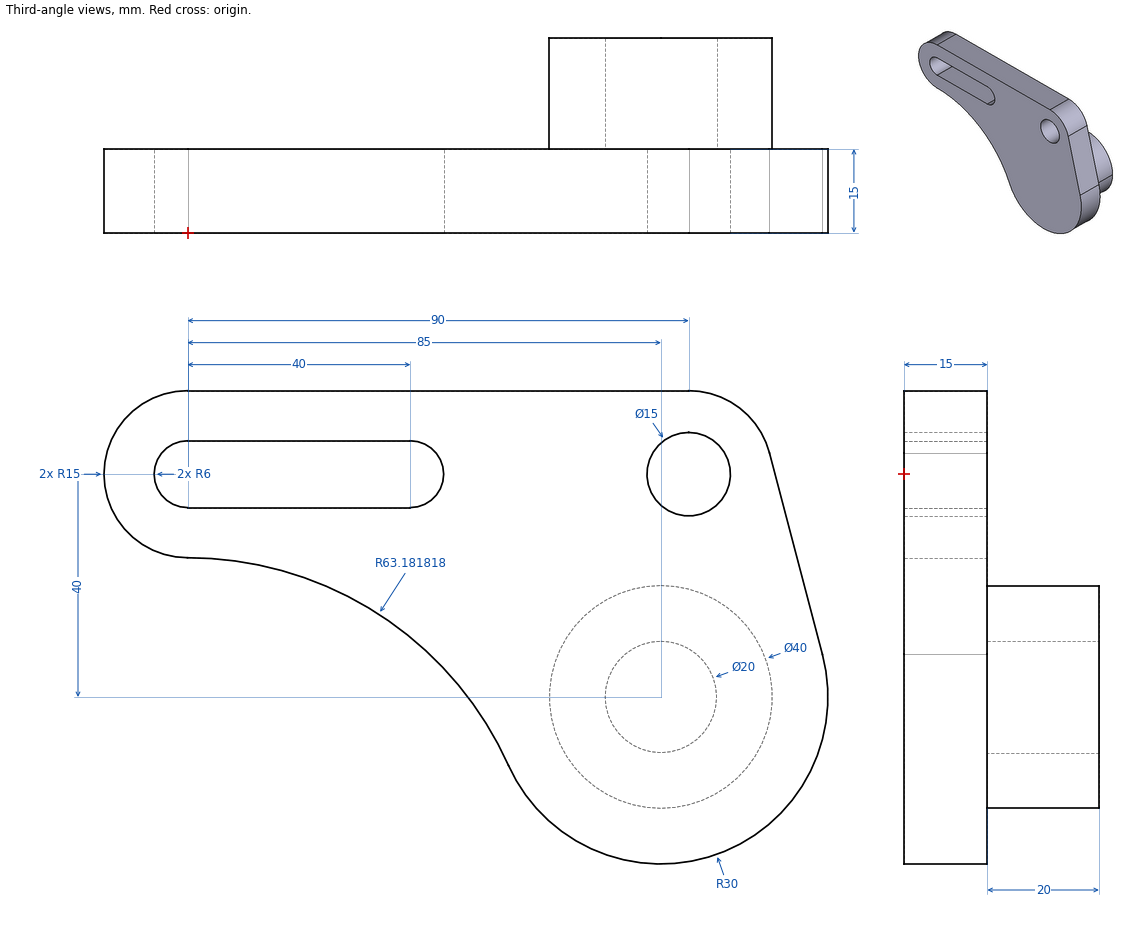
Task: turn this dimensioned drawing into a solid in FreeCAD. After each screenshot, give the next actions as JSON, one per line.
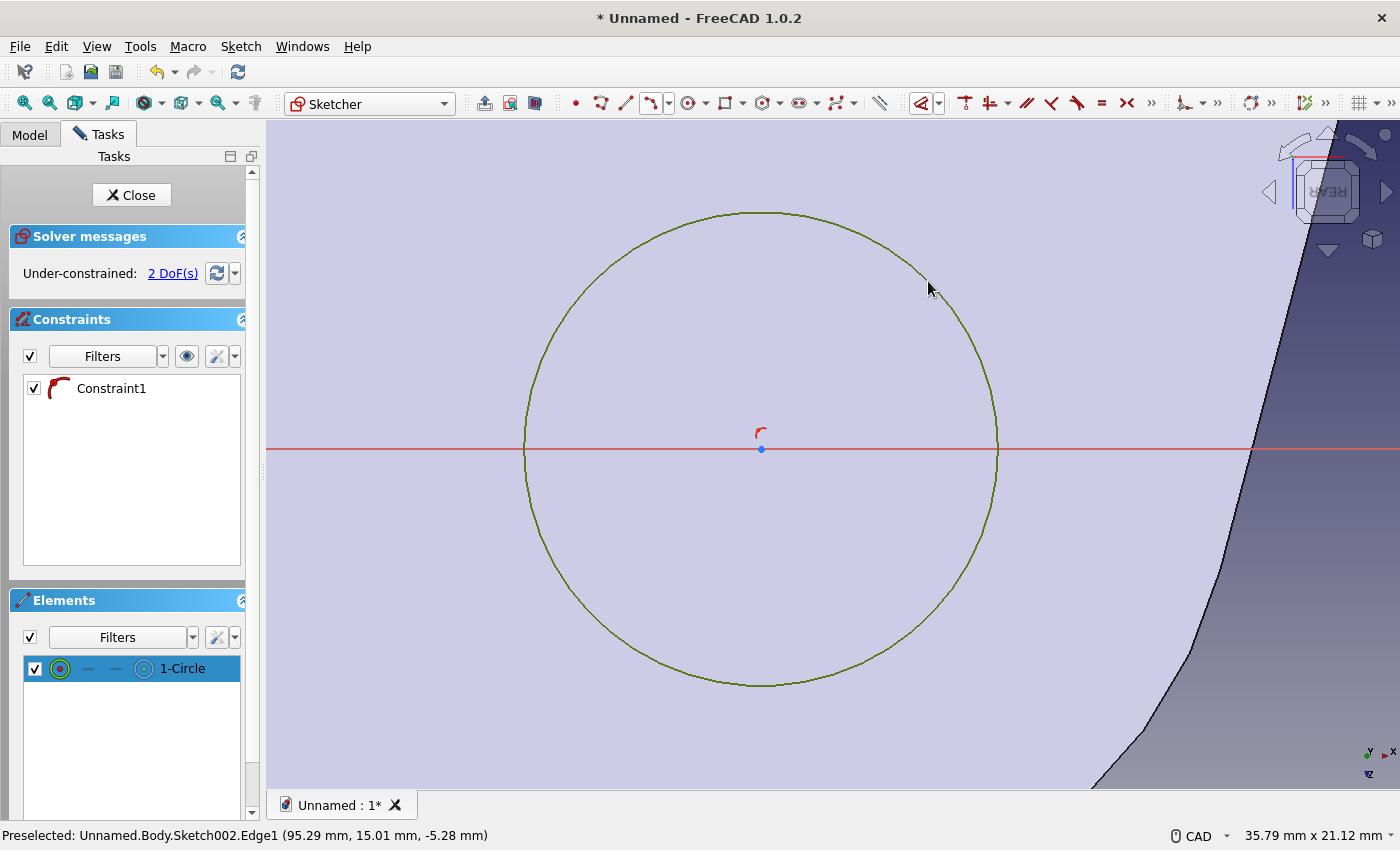
{"action": "left_click", "coordinate": [938, 104]}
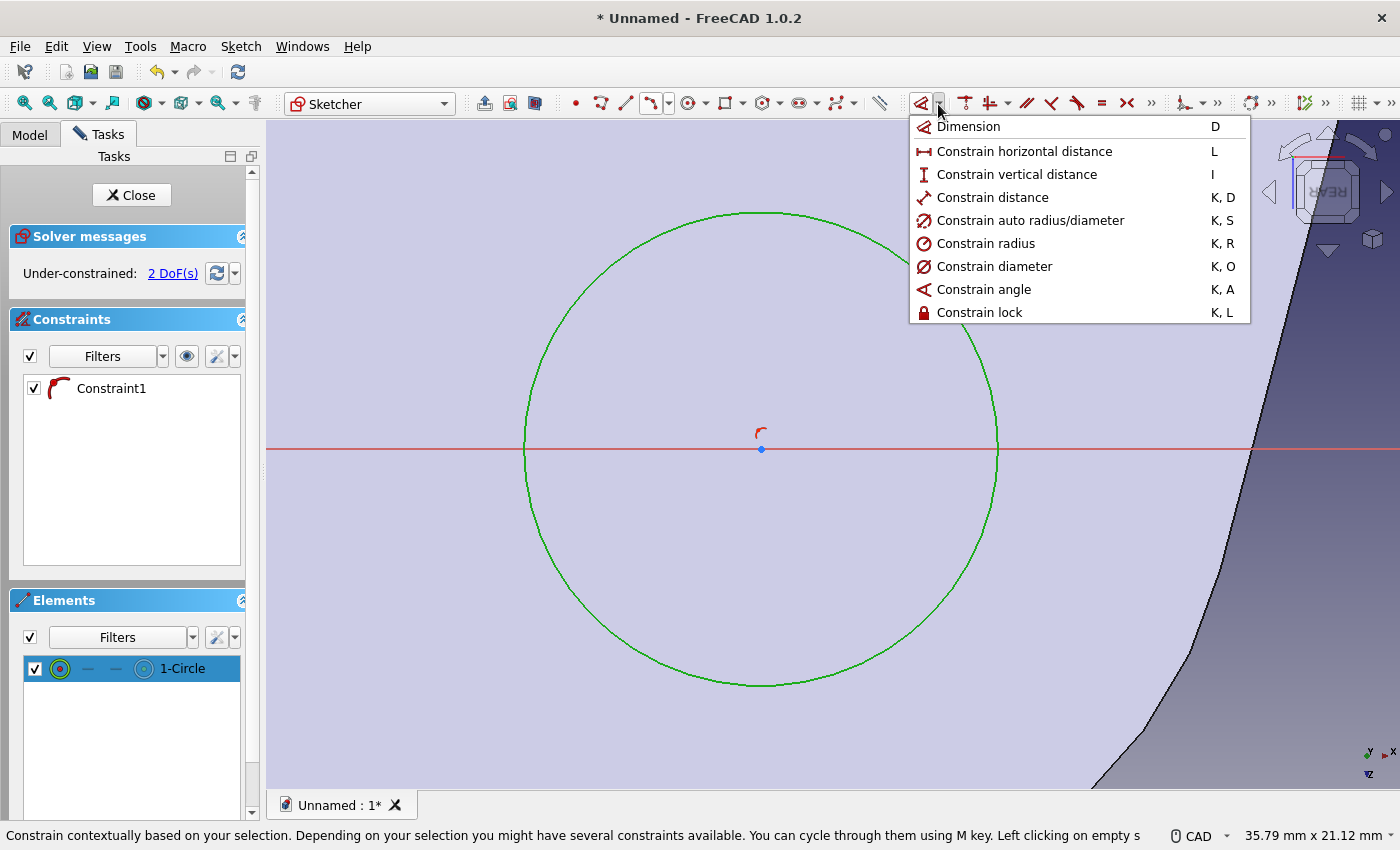
{"action": "left_click", "coordinate": [1080, 266]}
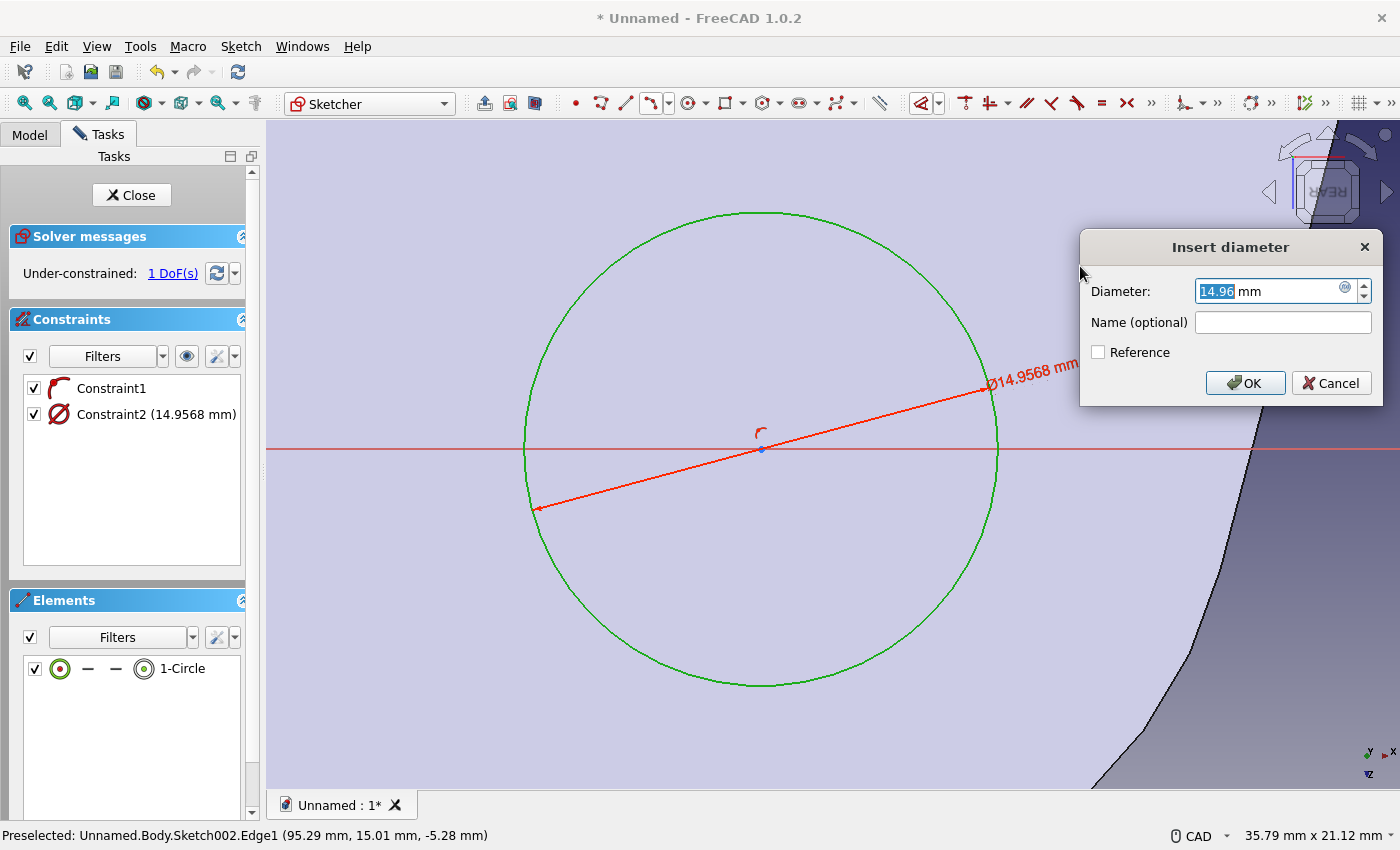
{"action": "type", "text": "15"}
{"action": "key", "text": "Return"}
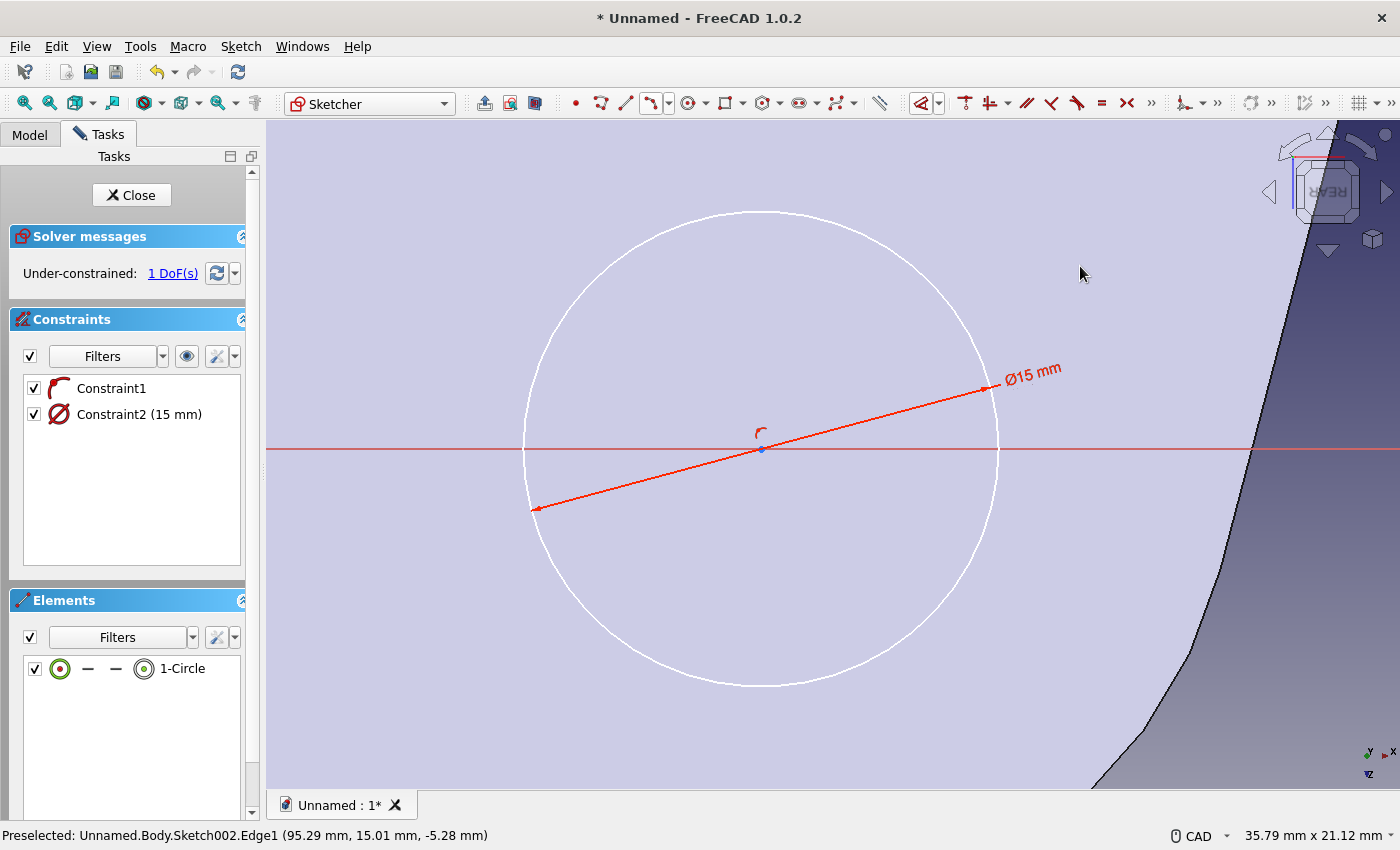
{"action": "left_click", "coordinate": [761, 449]}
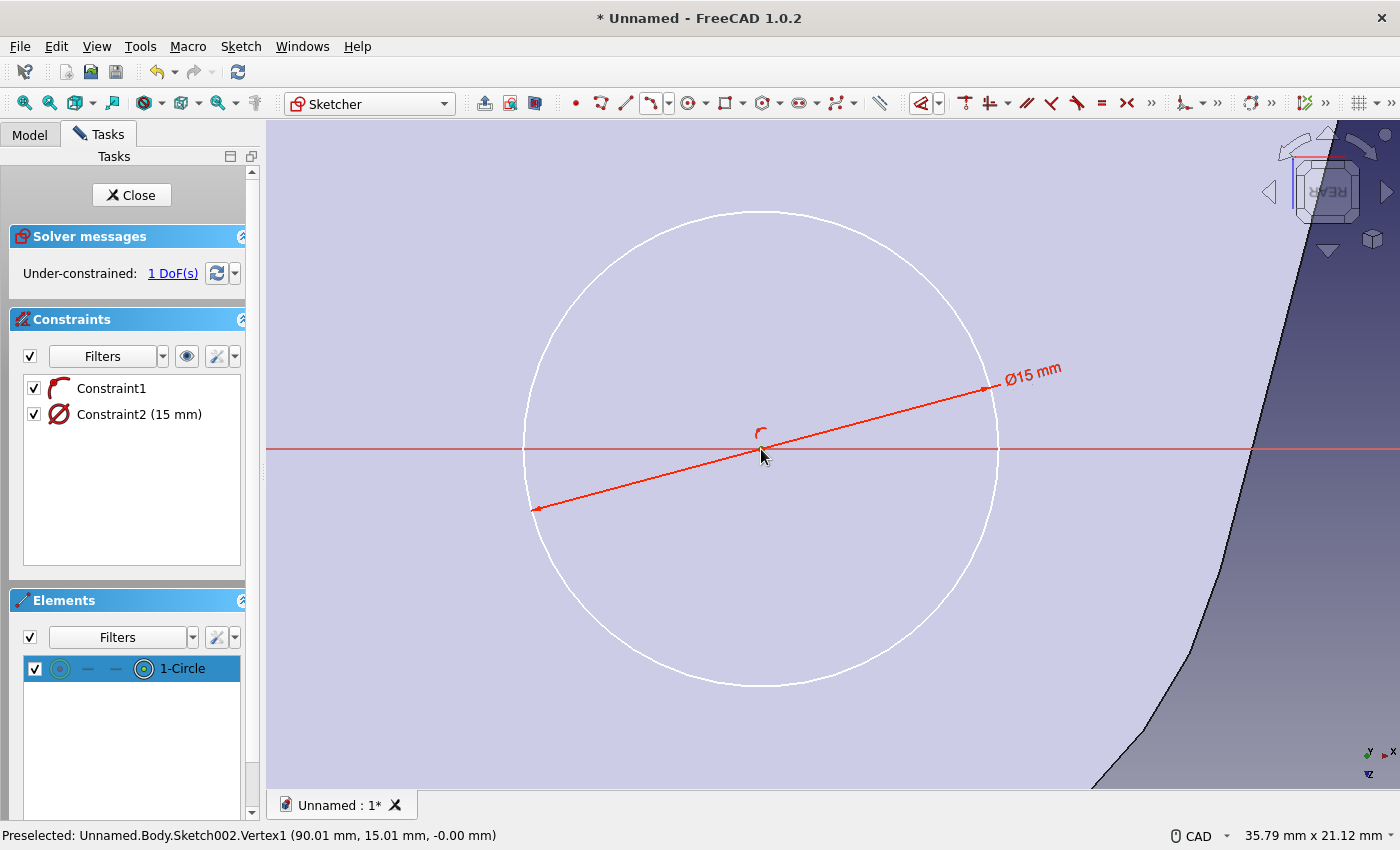
{"action": "left_click", "coordinate": [938, 104]}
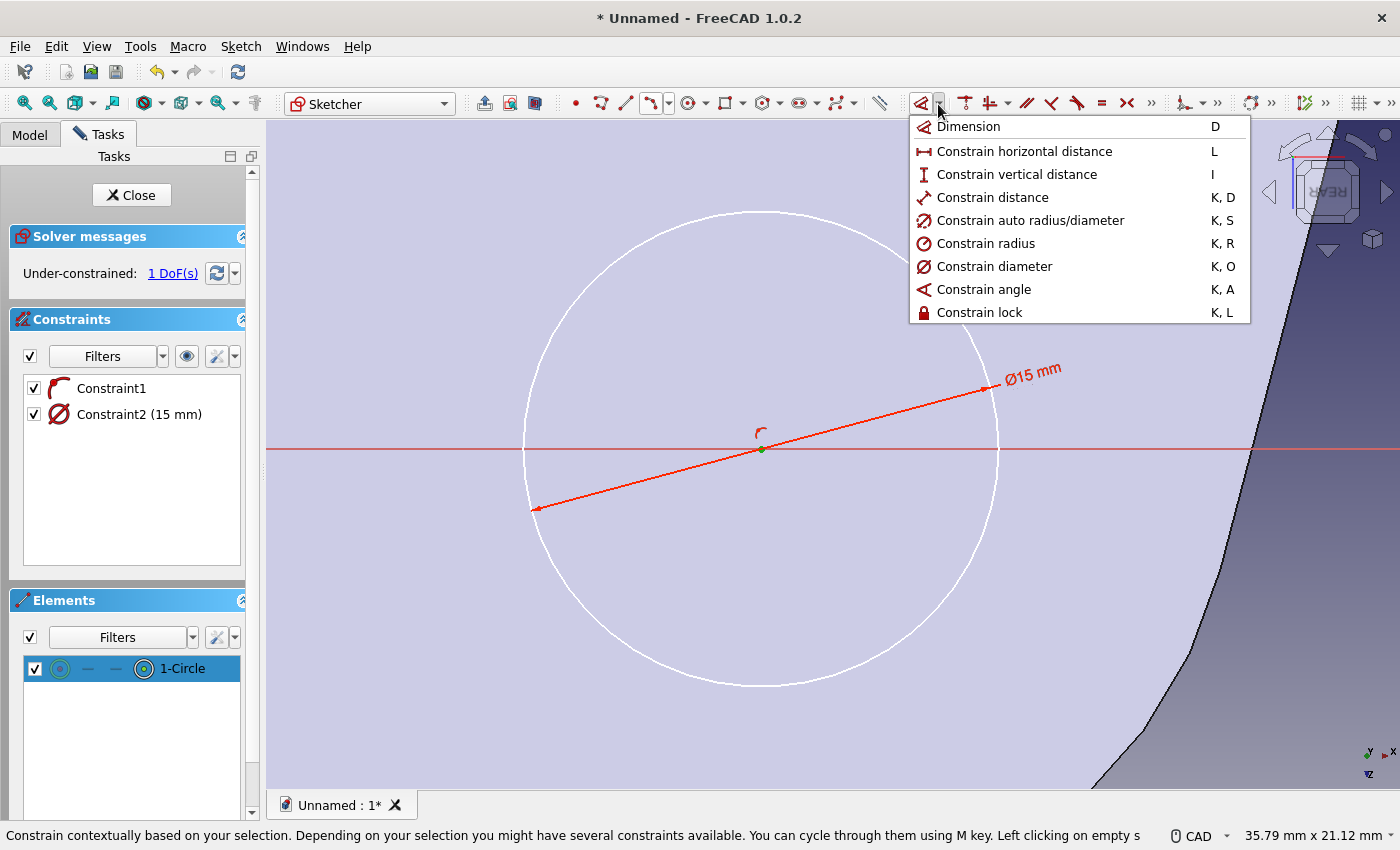
{"action": "left_click", "coordinate": [1080, 152]}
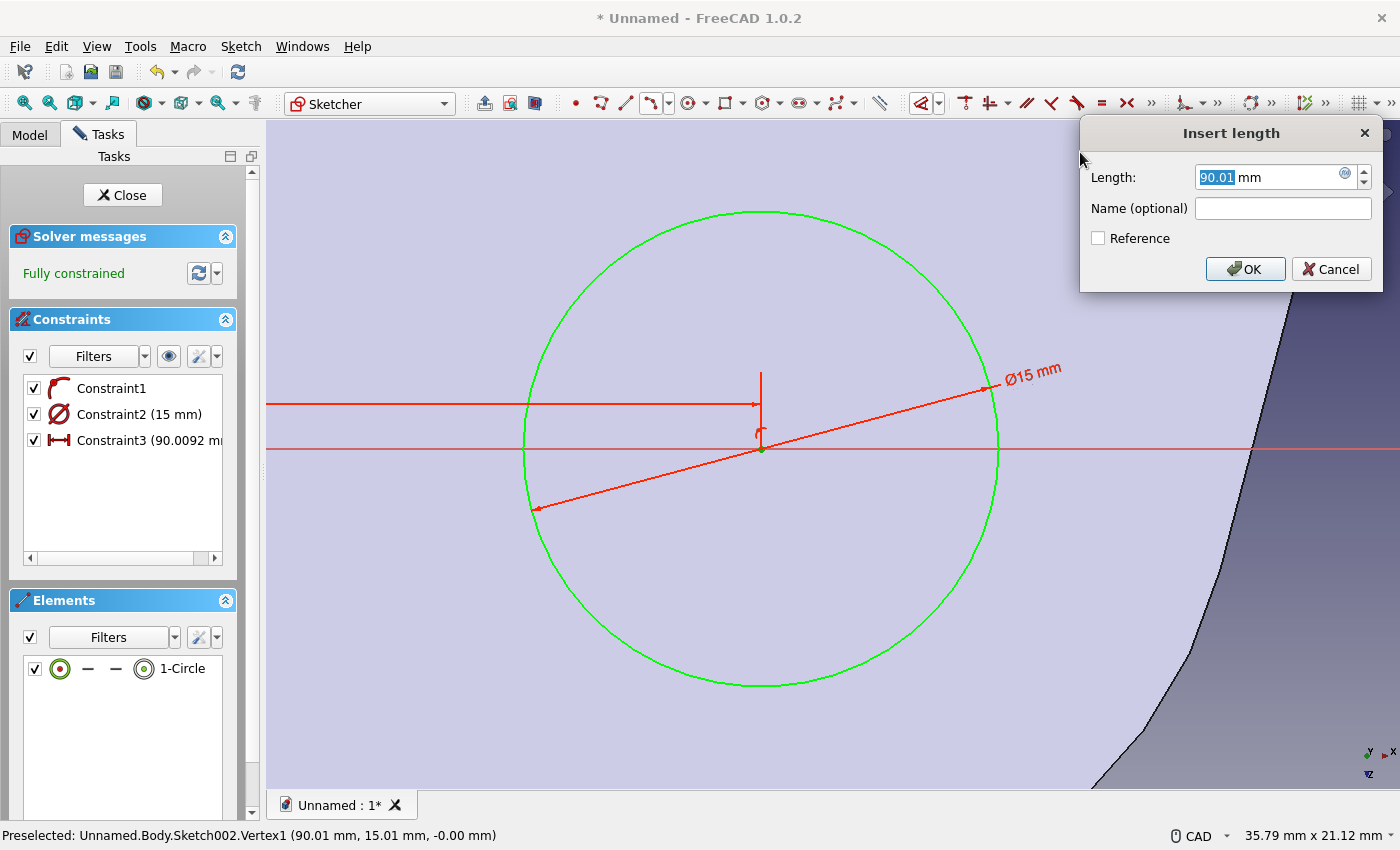
{"action": "type", "text": "90"}
{"action": "key", "text": "Return"}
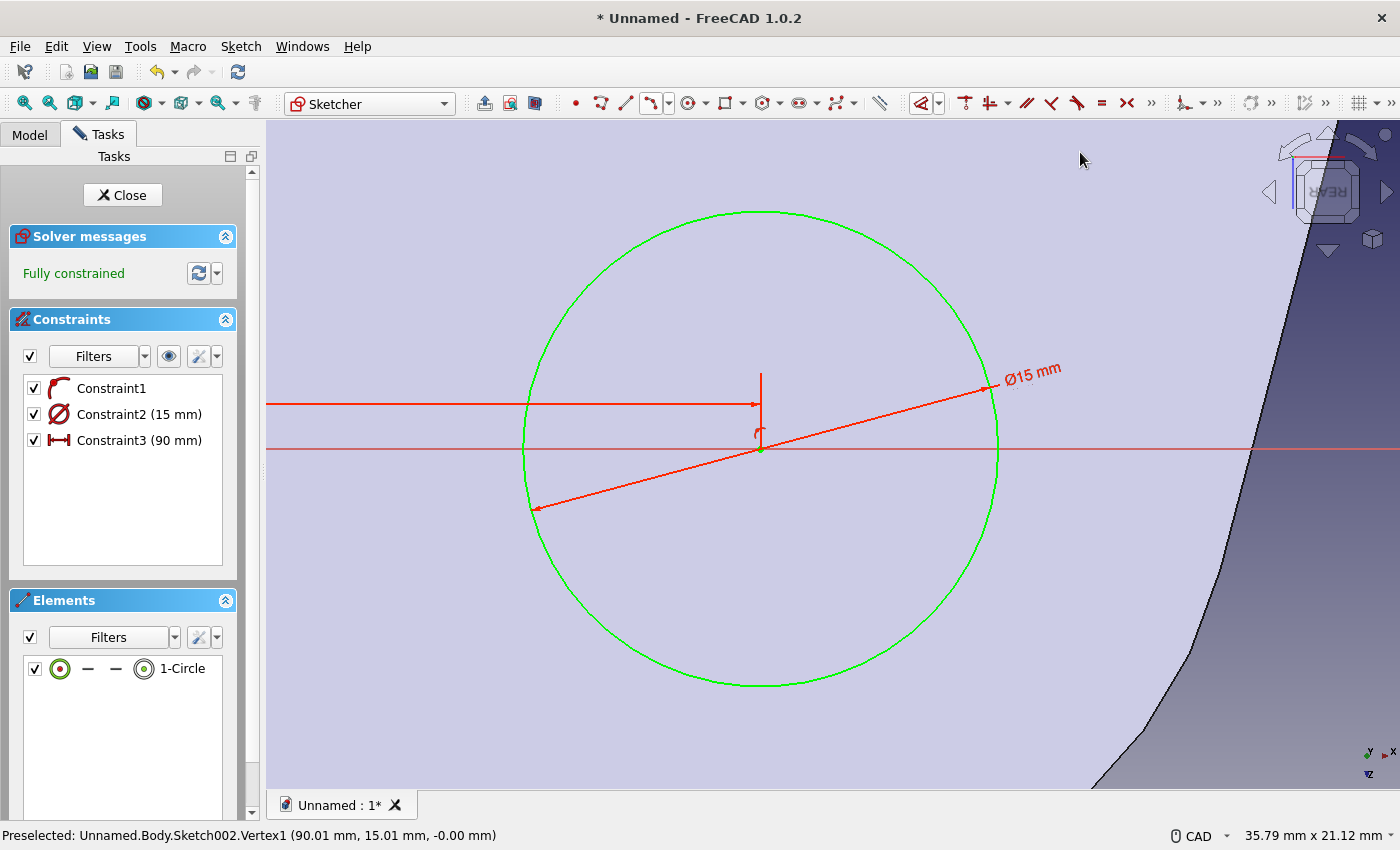
{"action": "left_click", "coordinate": [123, 195]}